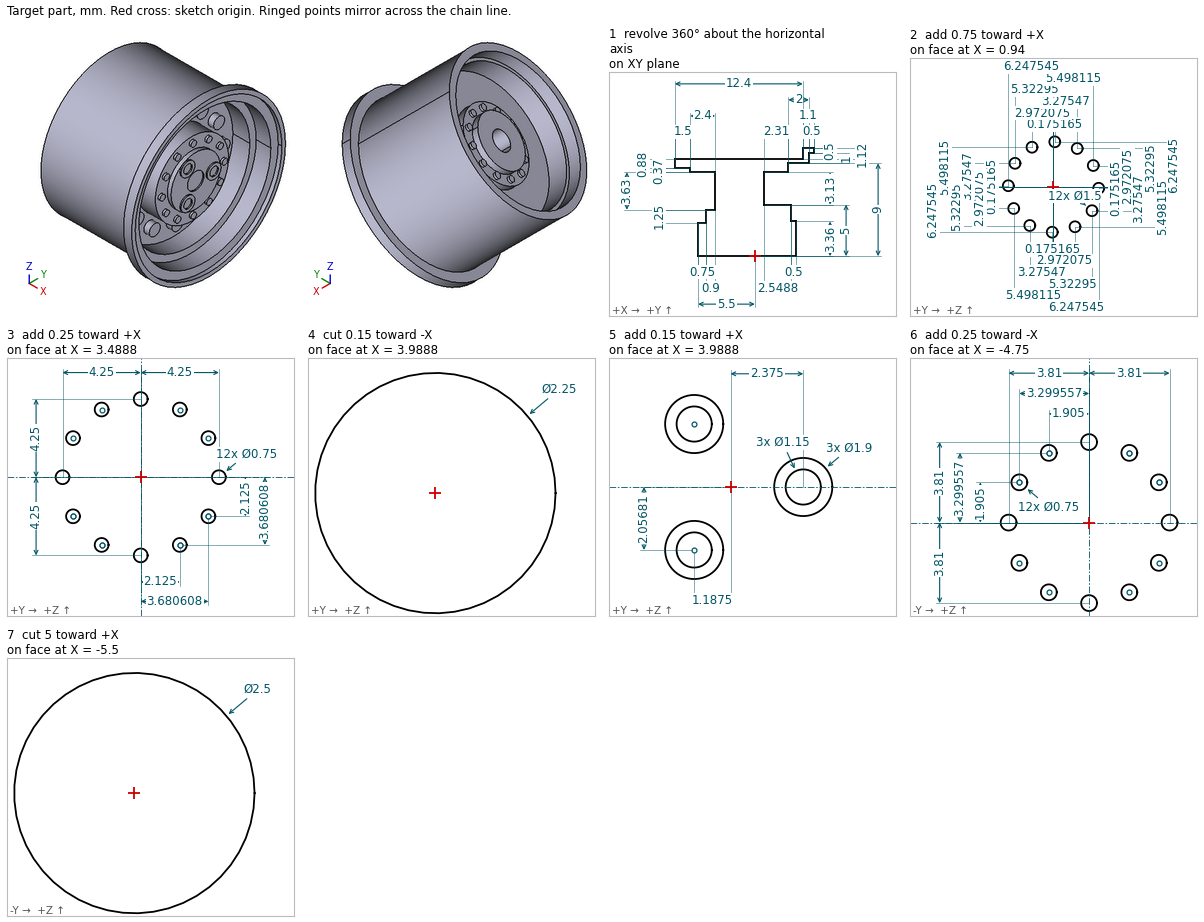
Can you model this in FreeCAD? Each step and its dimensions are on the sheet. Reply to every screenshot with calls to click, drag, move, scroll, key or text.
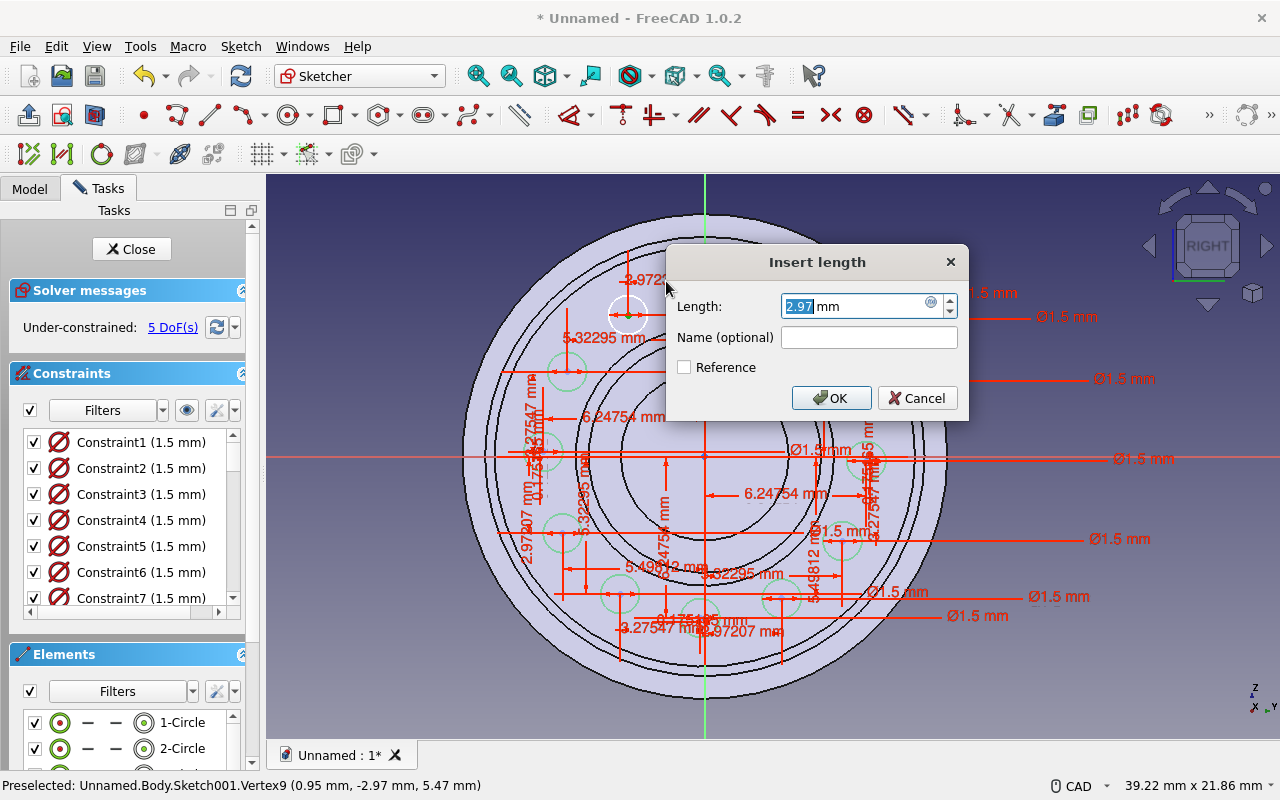
text(2.972075)
key(Return)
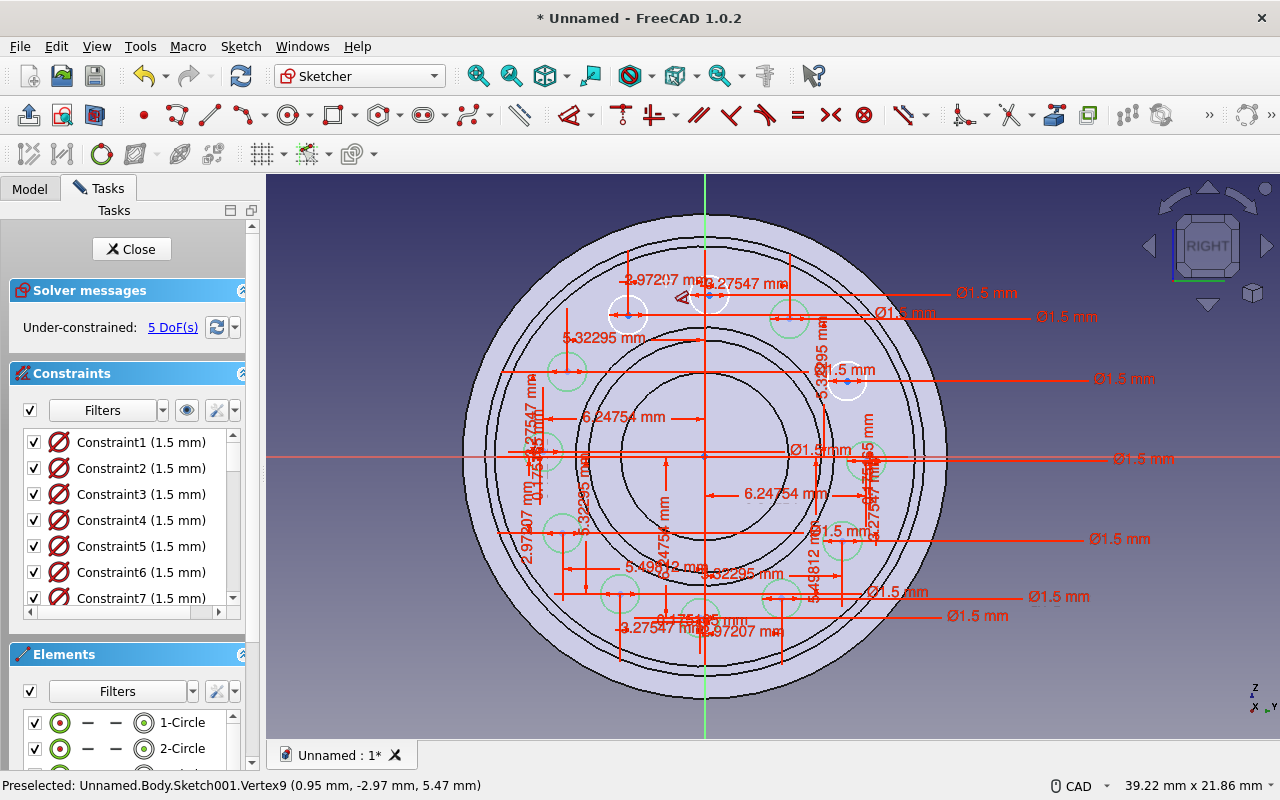
click(628, 315)
click(739, 386)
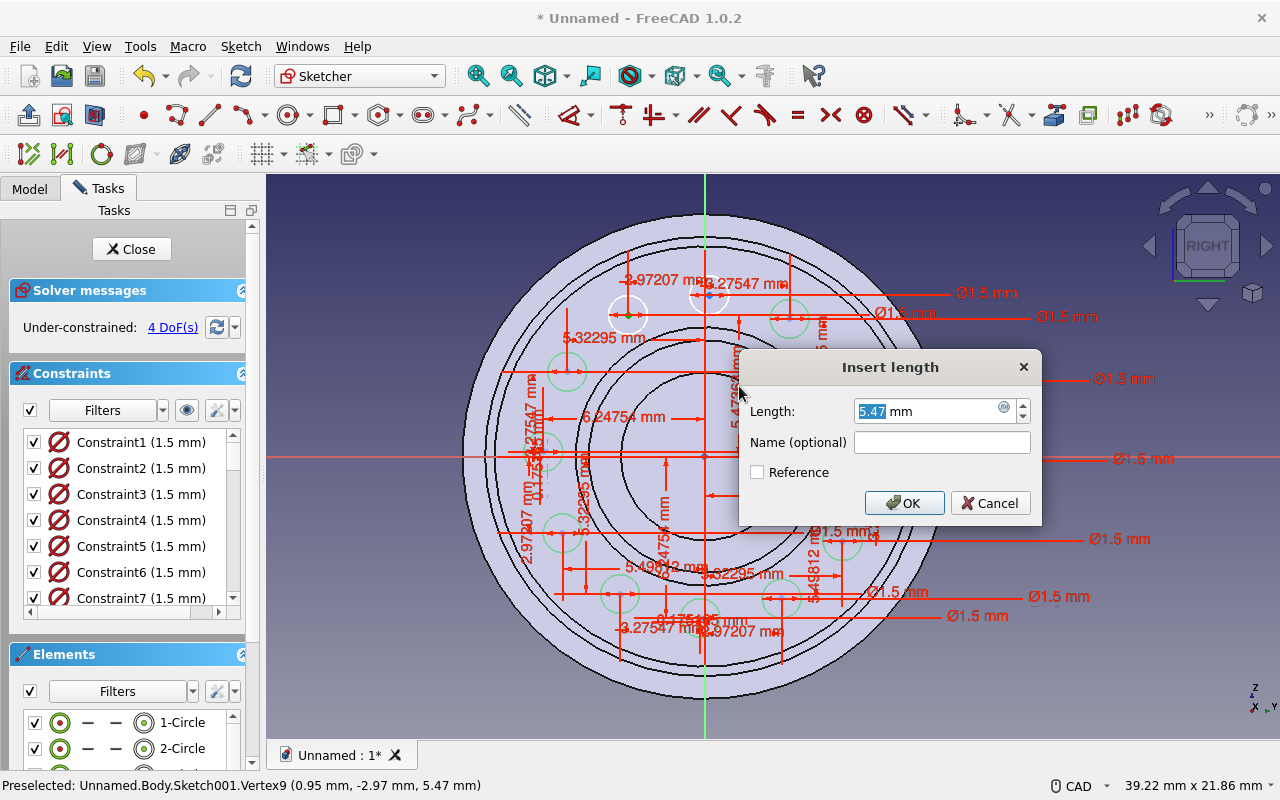
text(5.498115)
key(Return)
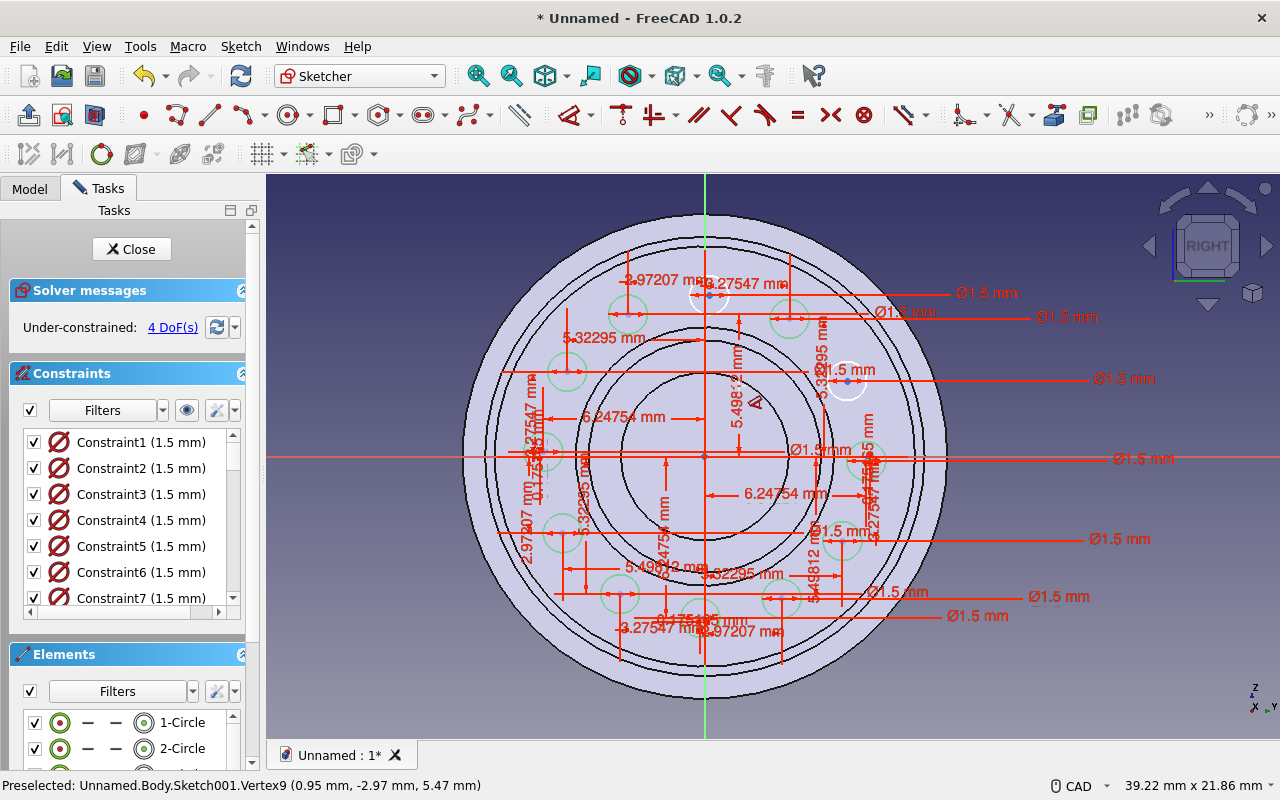
scroll(709, 295, up, 11)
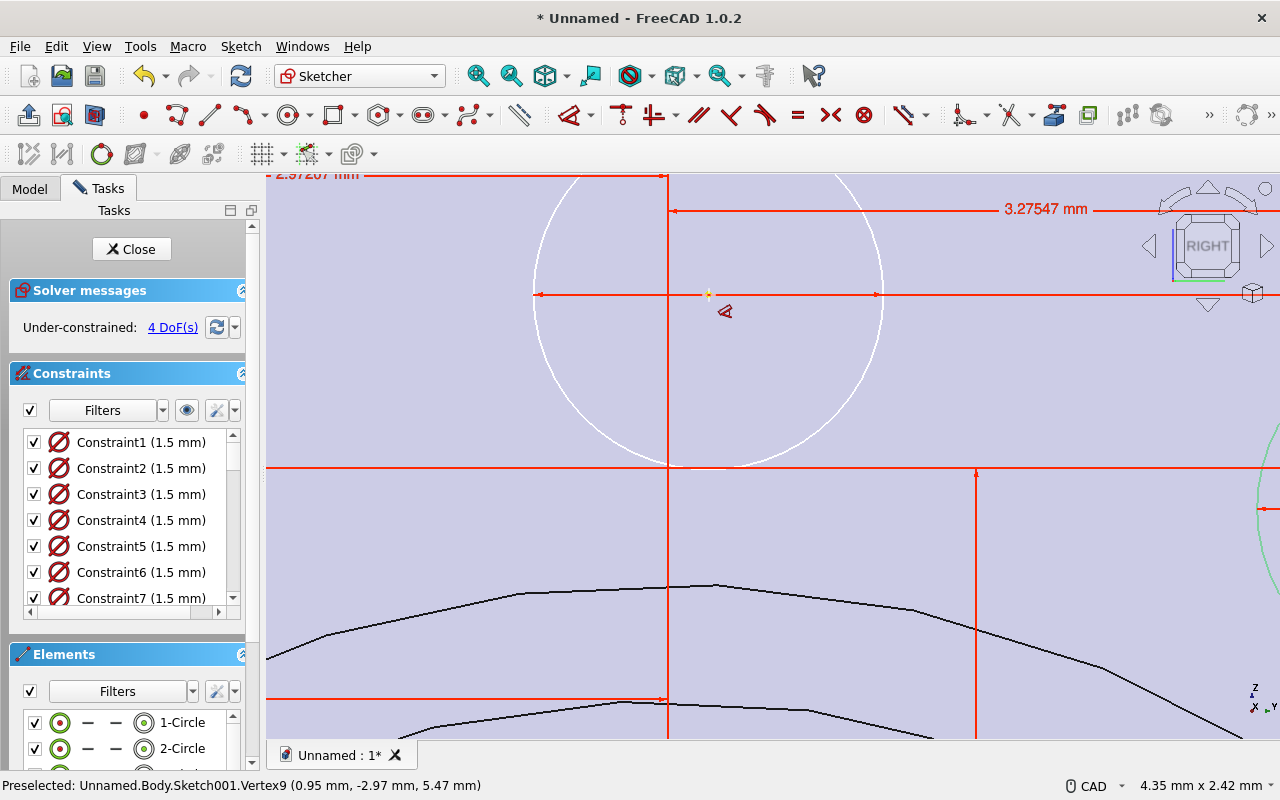
click(708, 295)
click(688, 261)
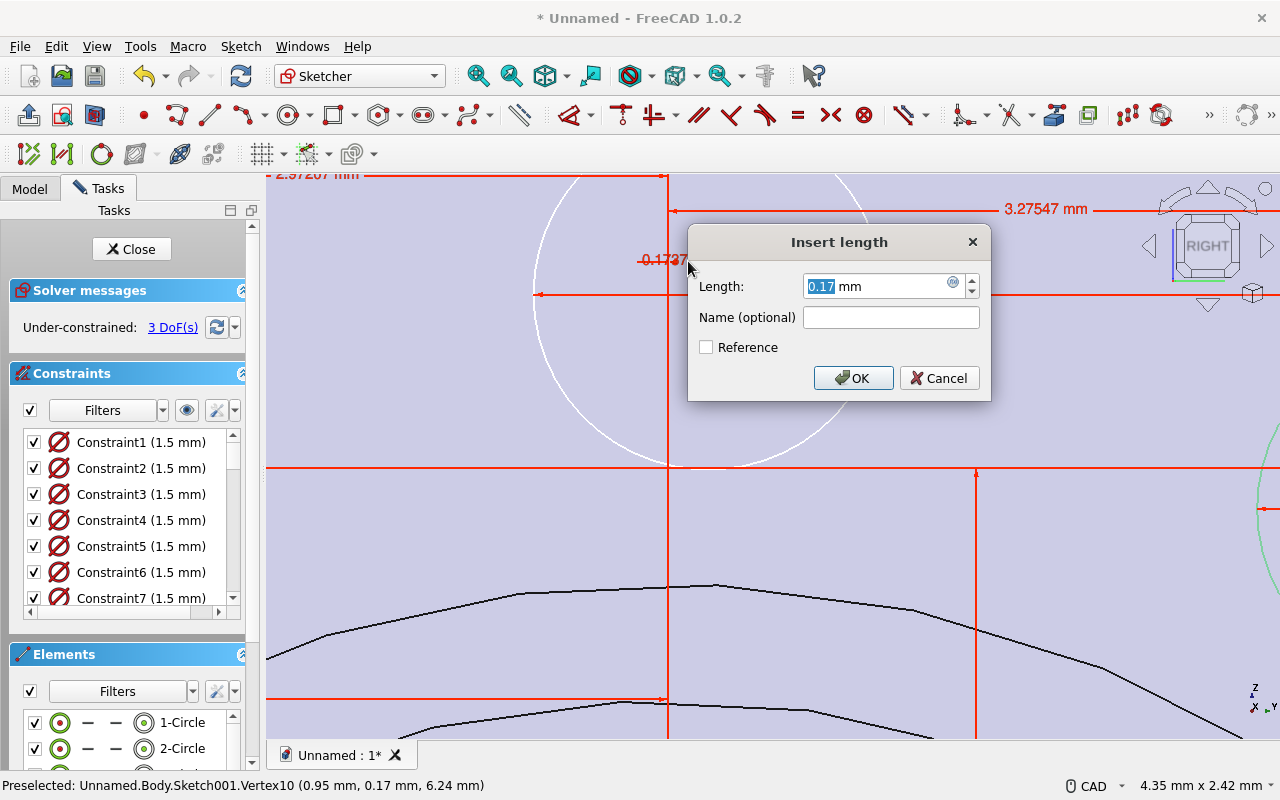
text(0.175165)
key(Return)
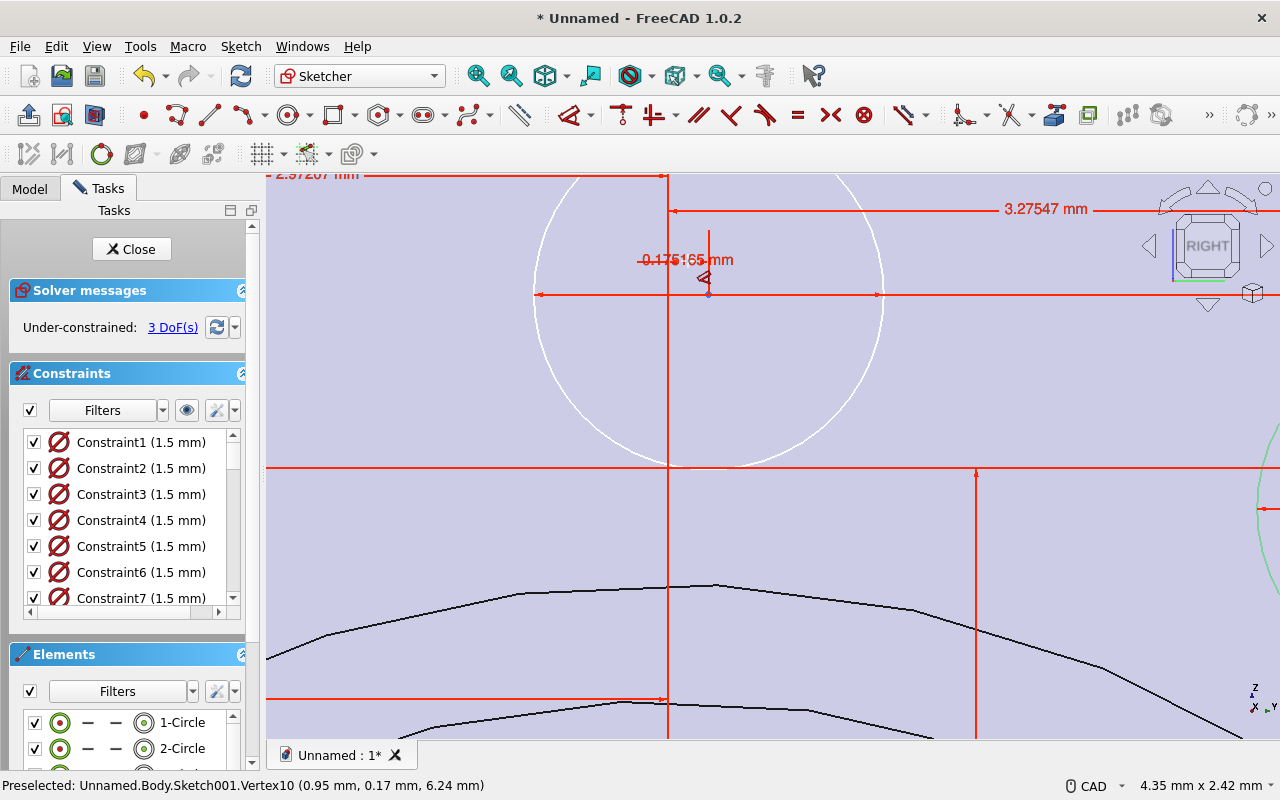
scroll(709, 295, down, 11)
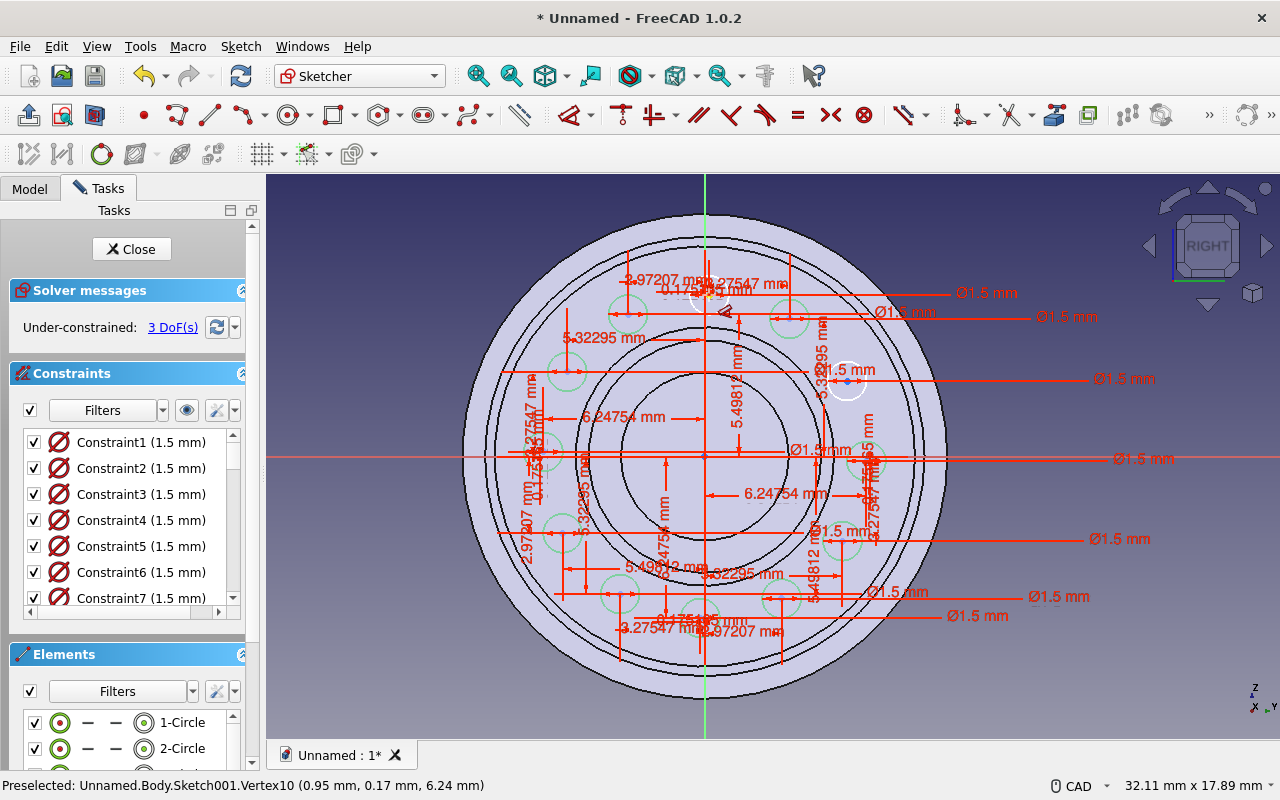
click(709, 295)
click(743, 339)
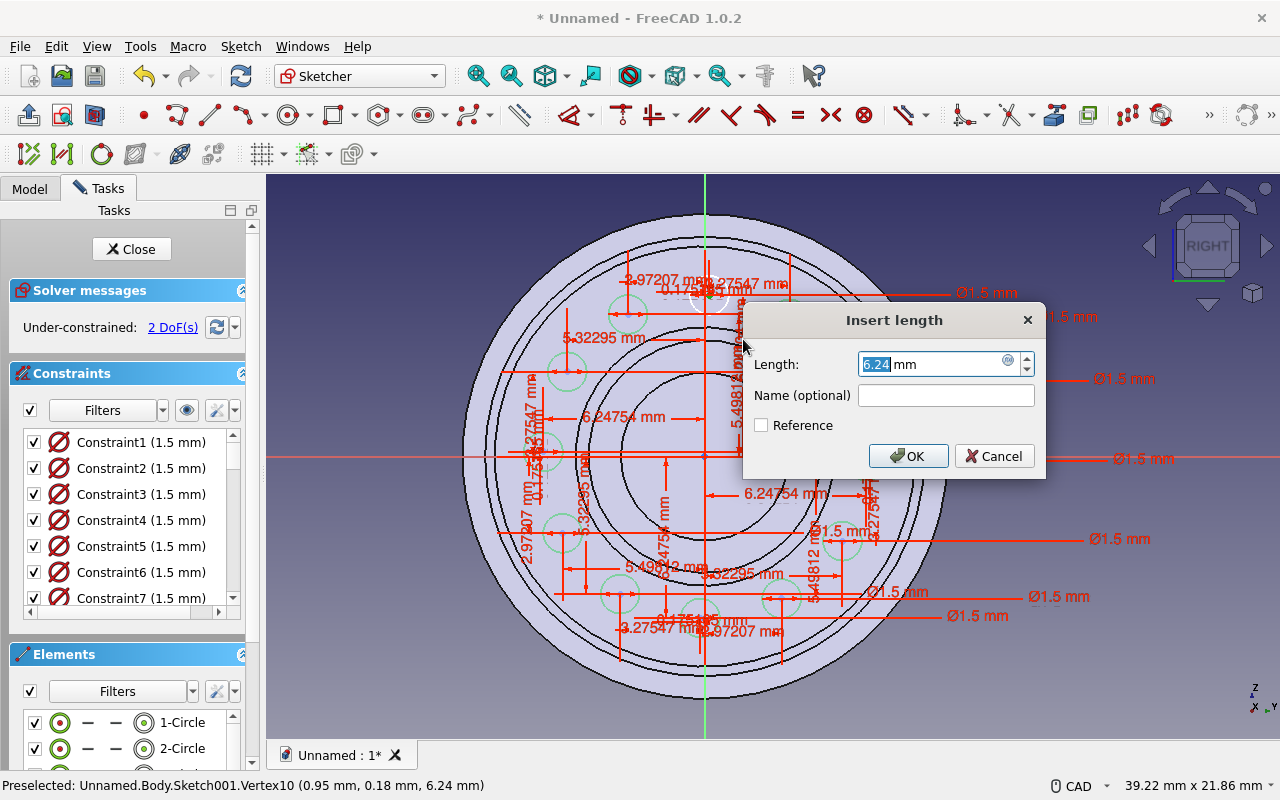
text(6.247545)
key(Return)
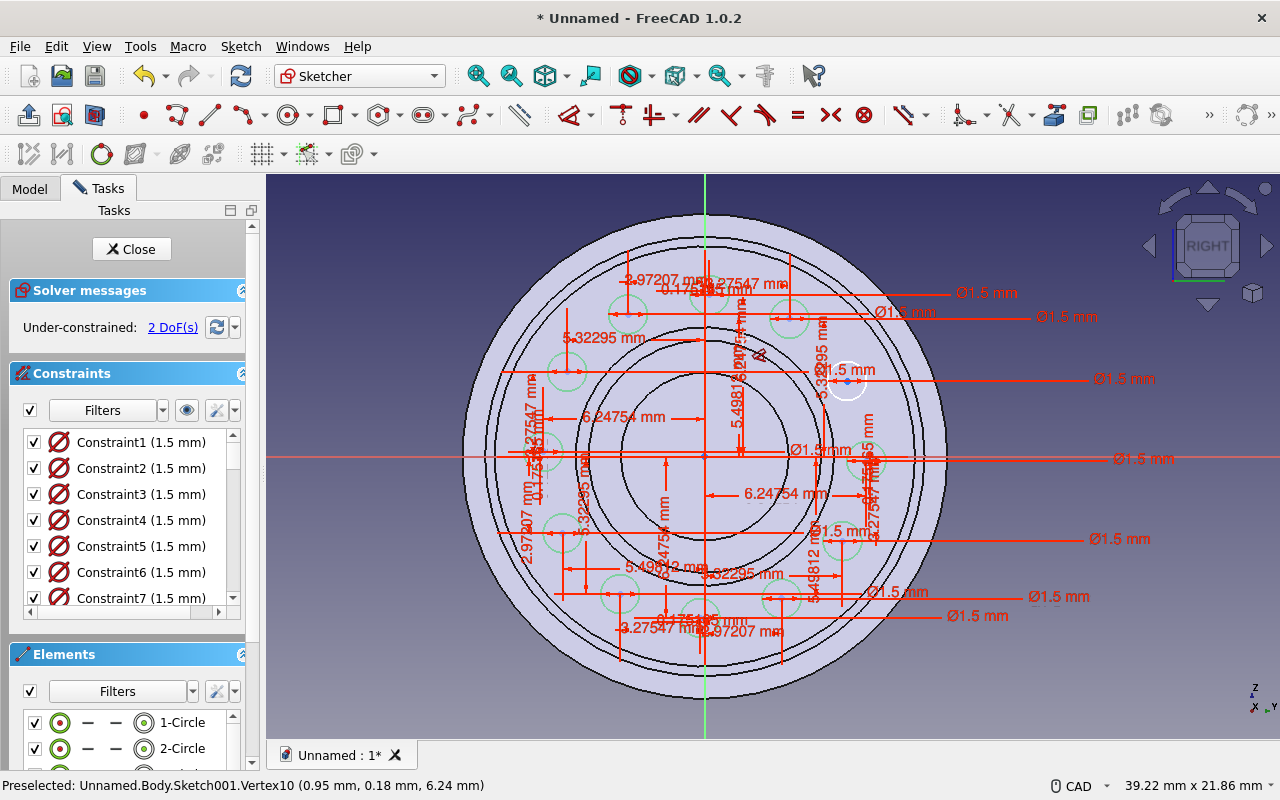
click(847, 381)
click(826, 323)